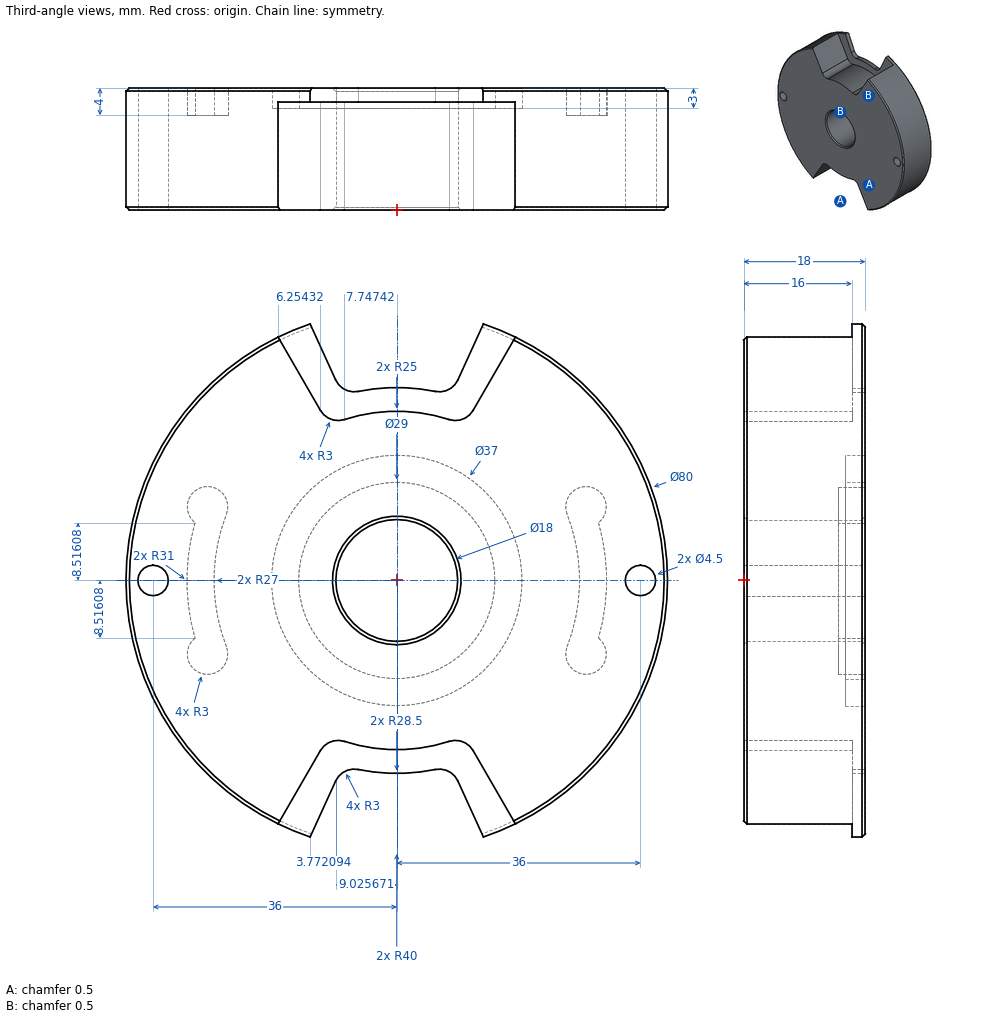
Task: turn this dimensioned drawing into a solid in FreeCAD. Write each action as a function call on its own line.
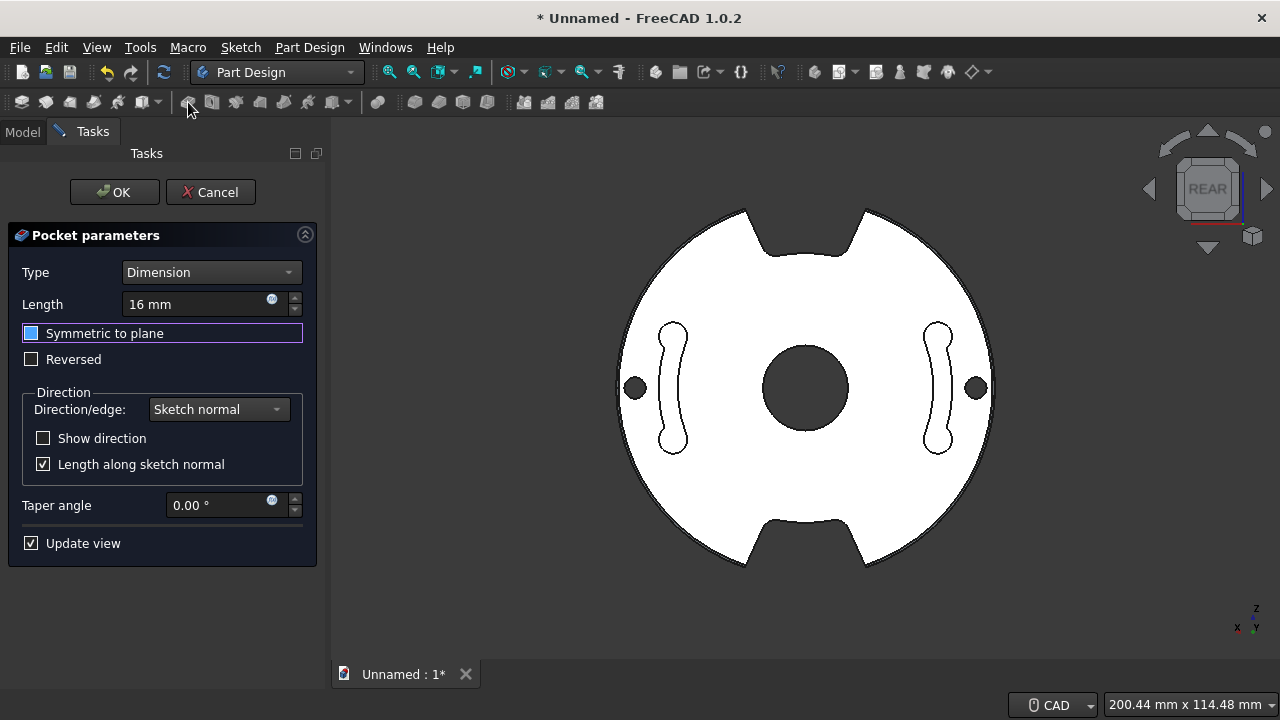
click(115, 192)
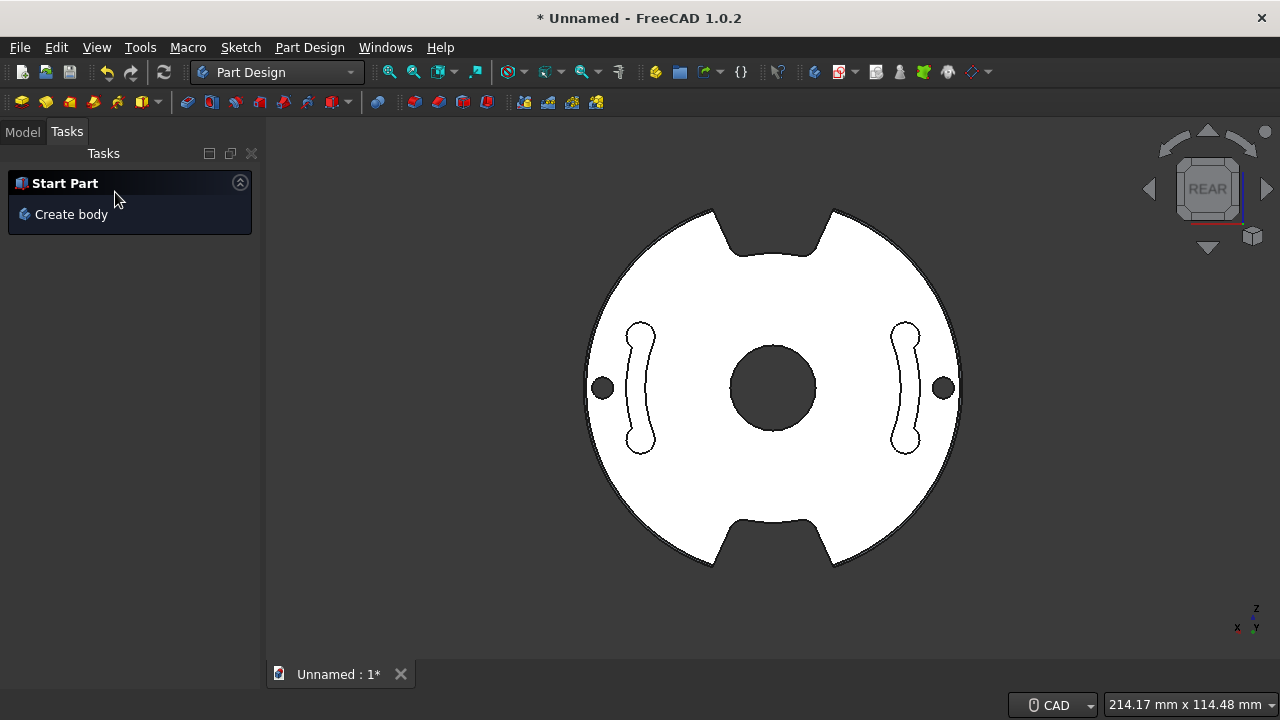
click(666, 488)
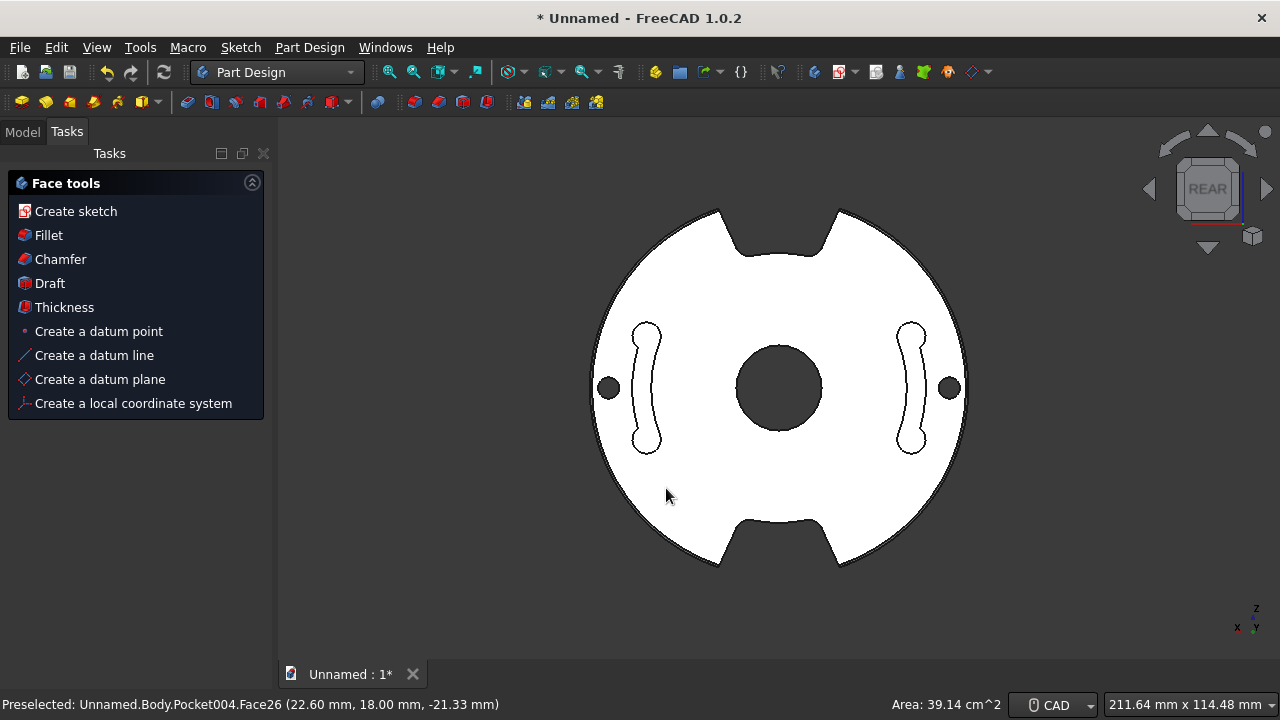
click(840, 72)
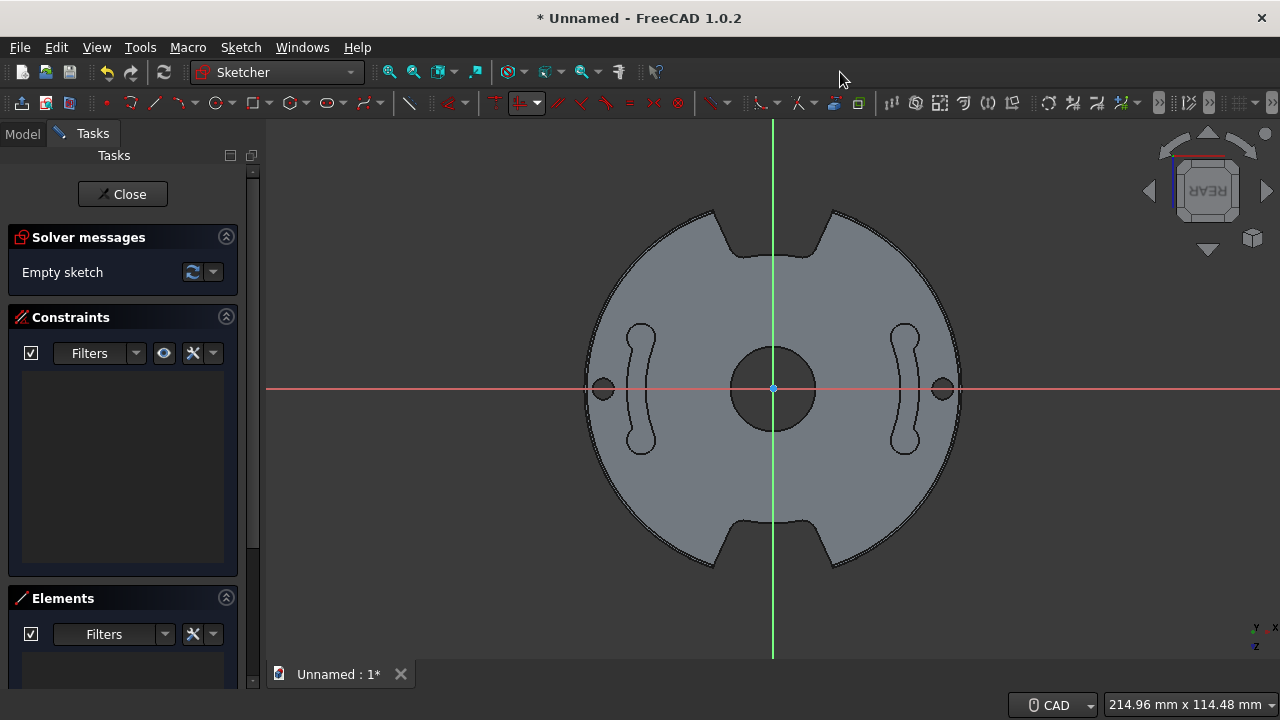
scroll(856, 389, up, 3)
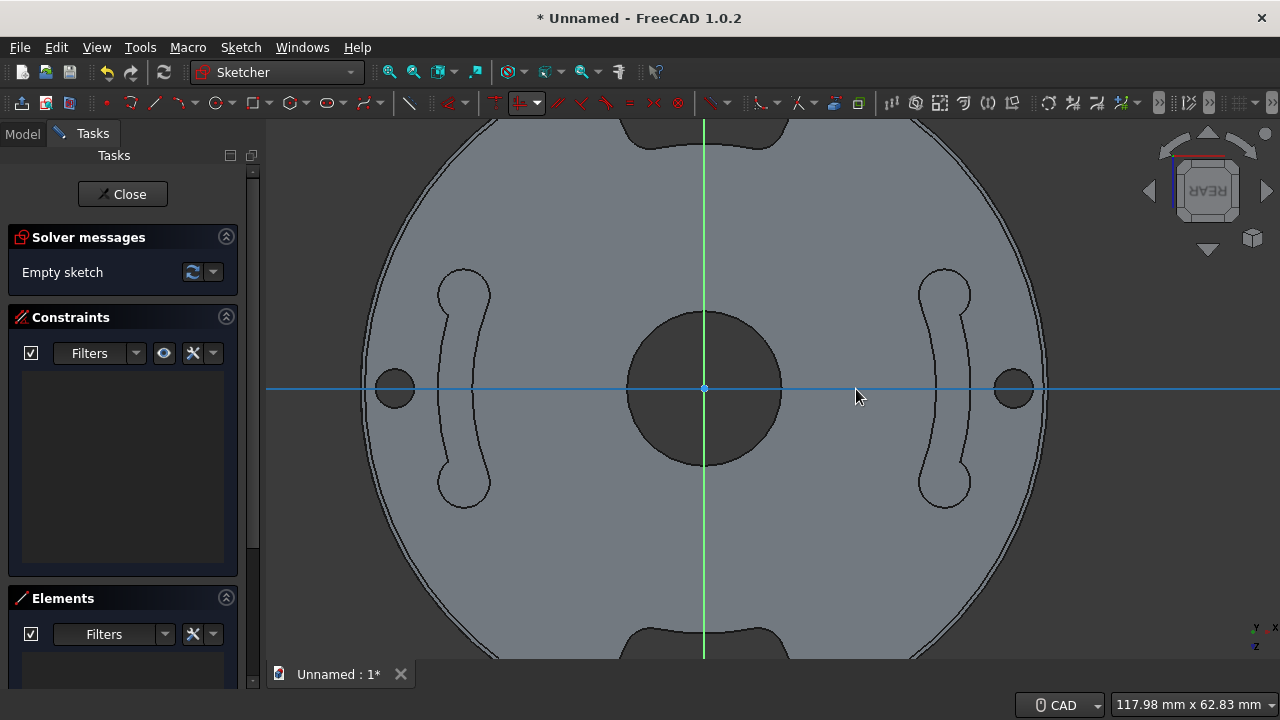
click(216, 104)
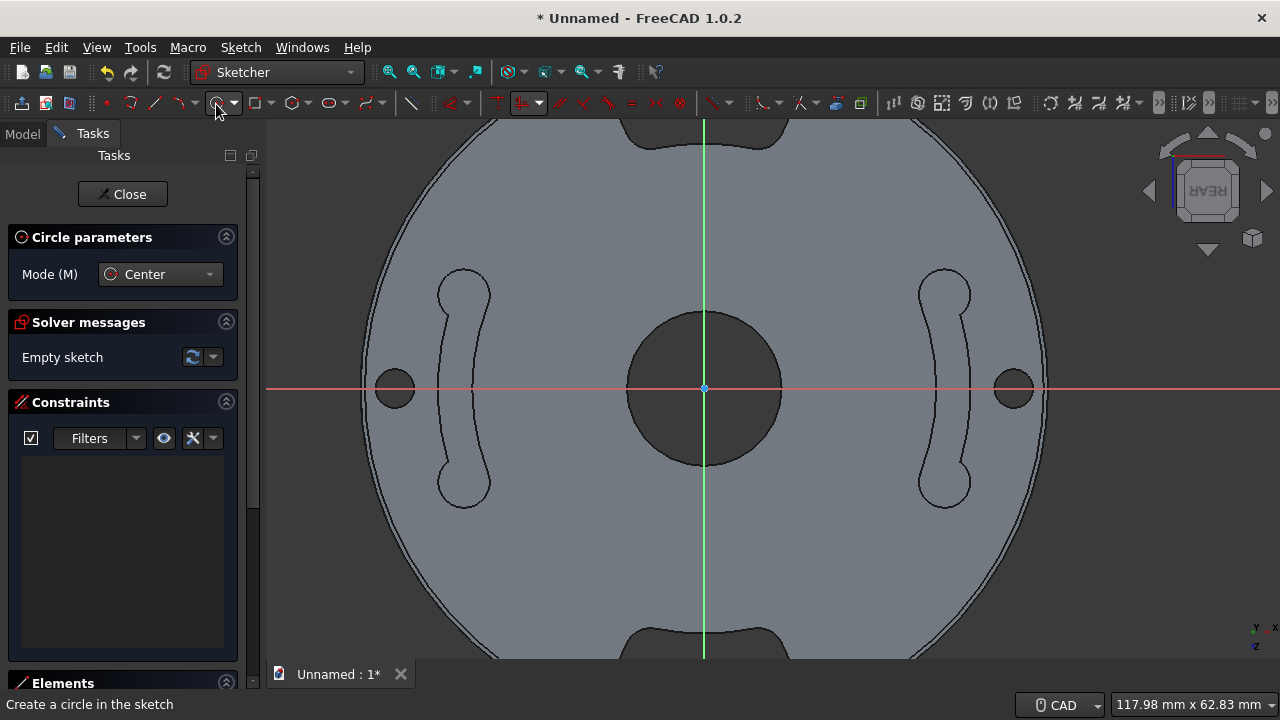
click(704, 389)
click(817, 276)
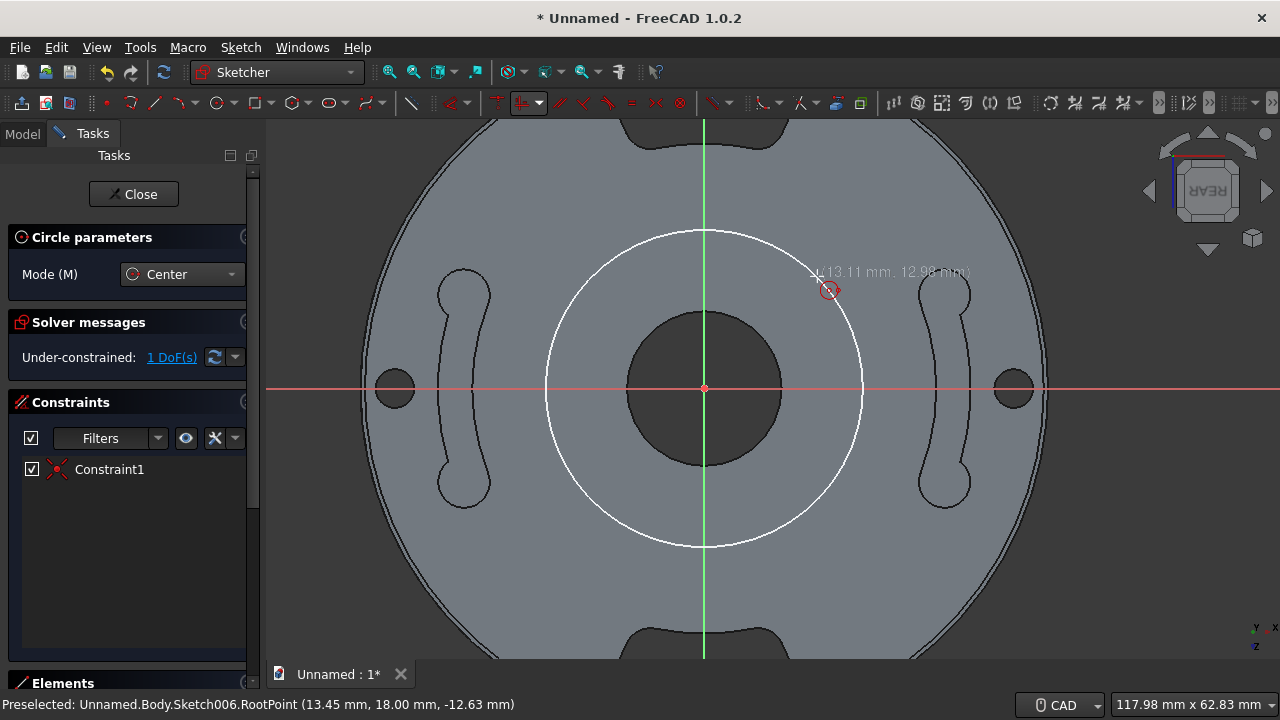
click(704, 389)
click(792, 300)
key(Escape)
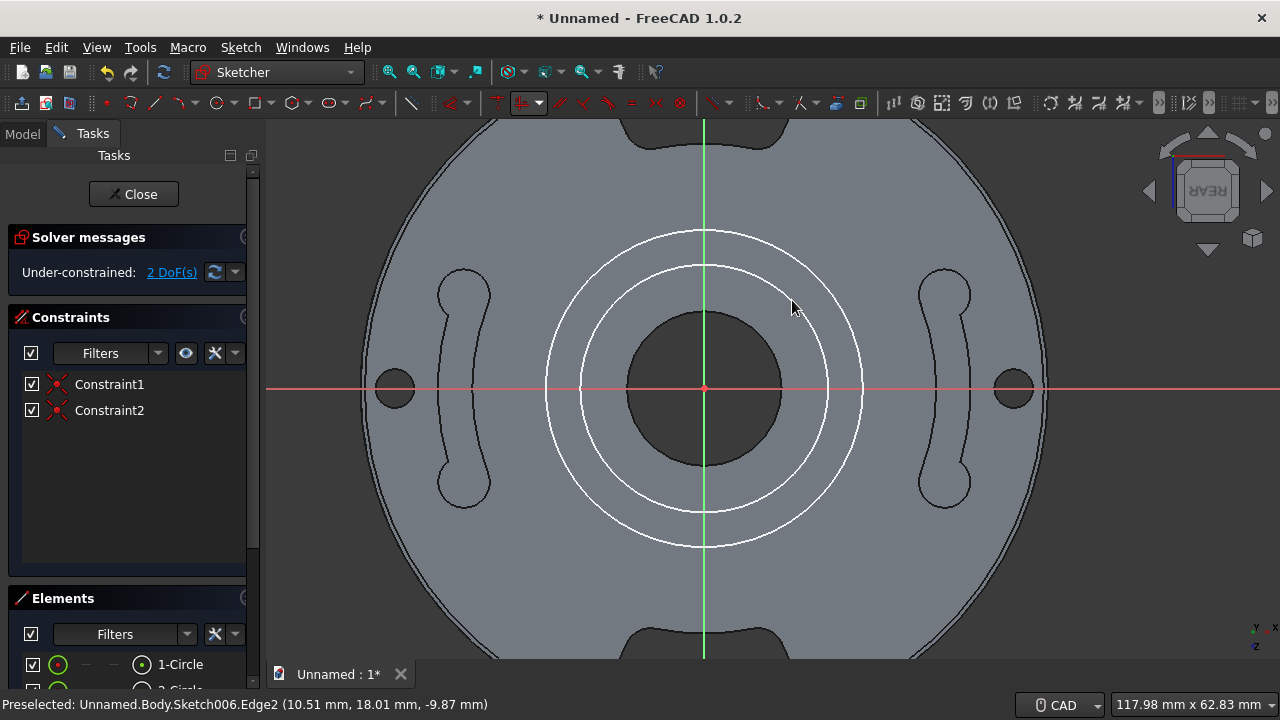
click(450, 104)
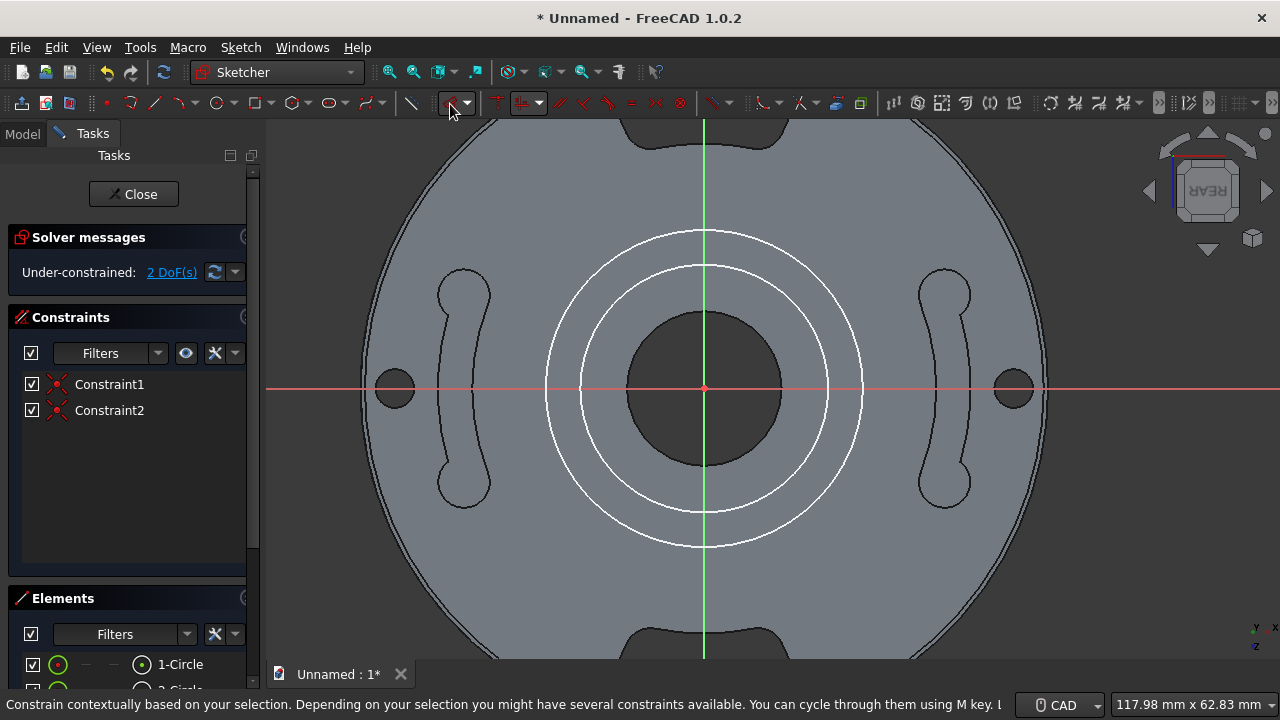
click(816, 276)
click(839, 253)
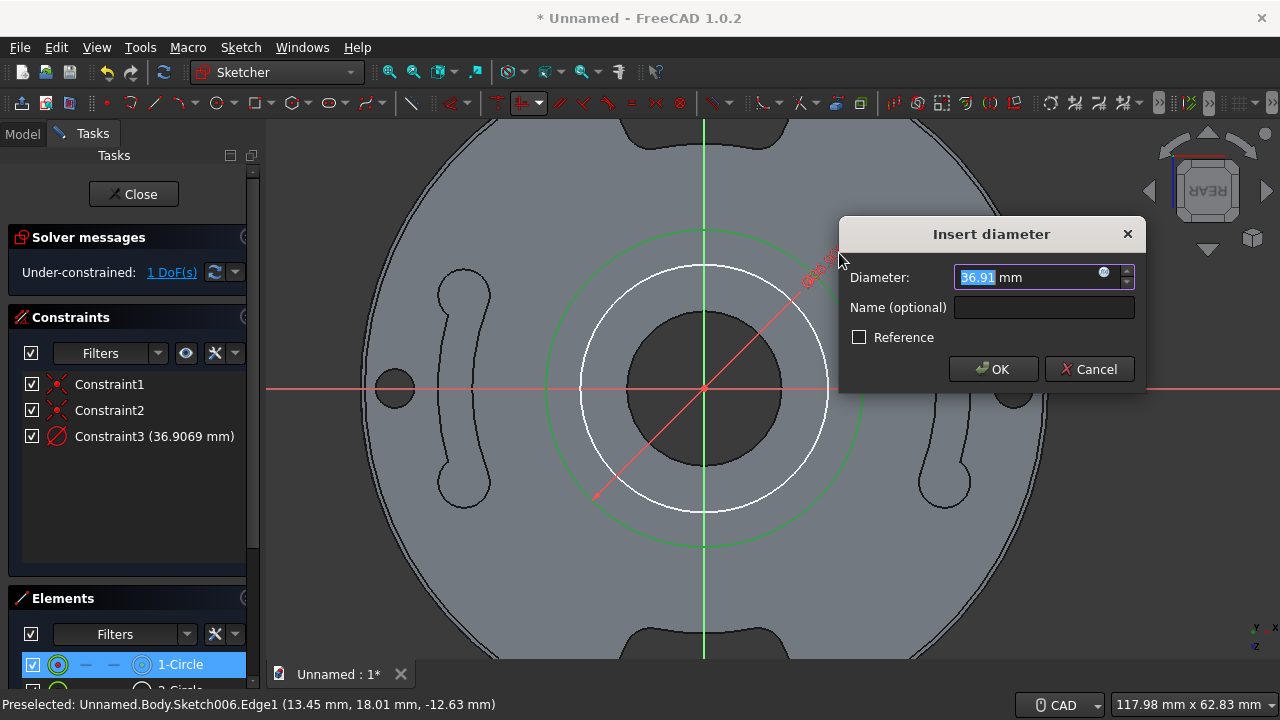
text(37)
key(Return)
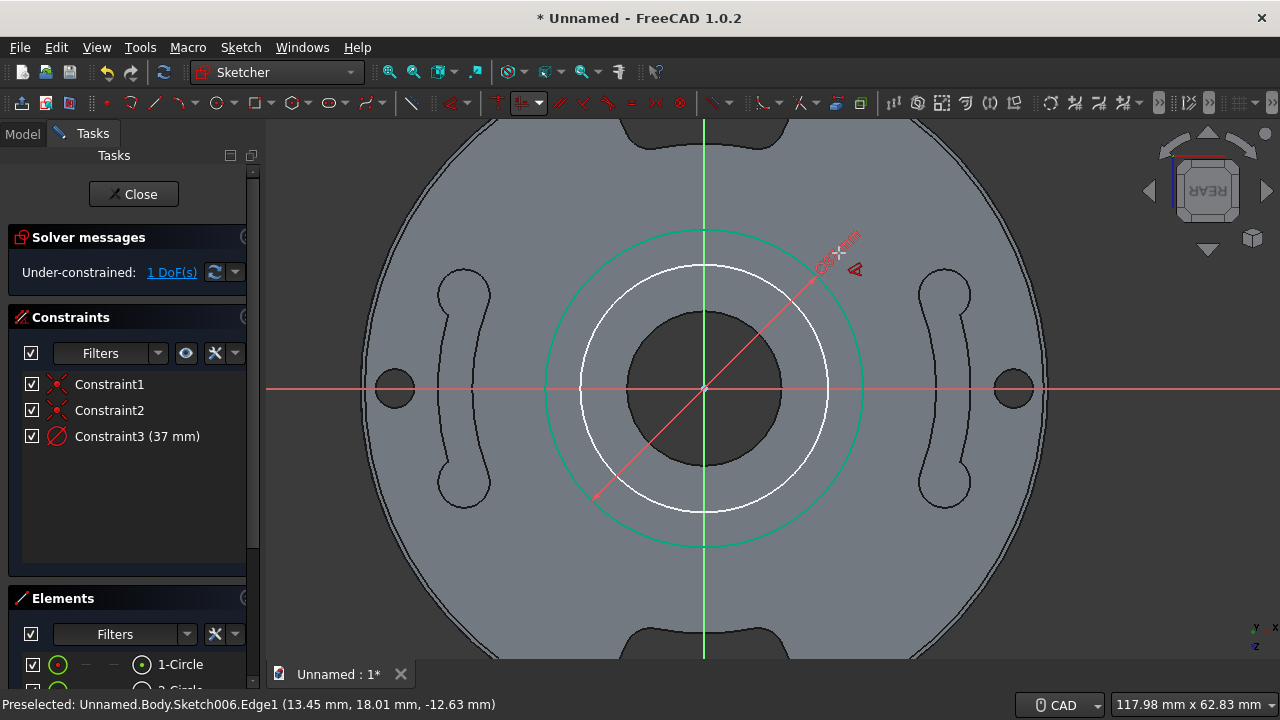
click(792, 301)
click(876, 338)